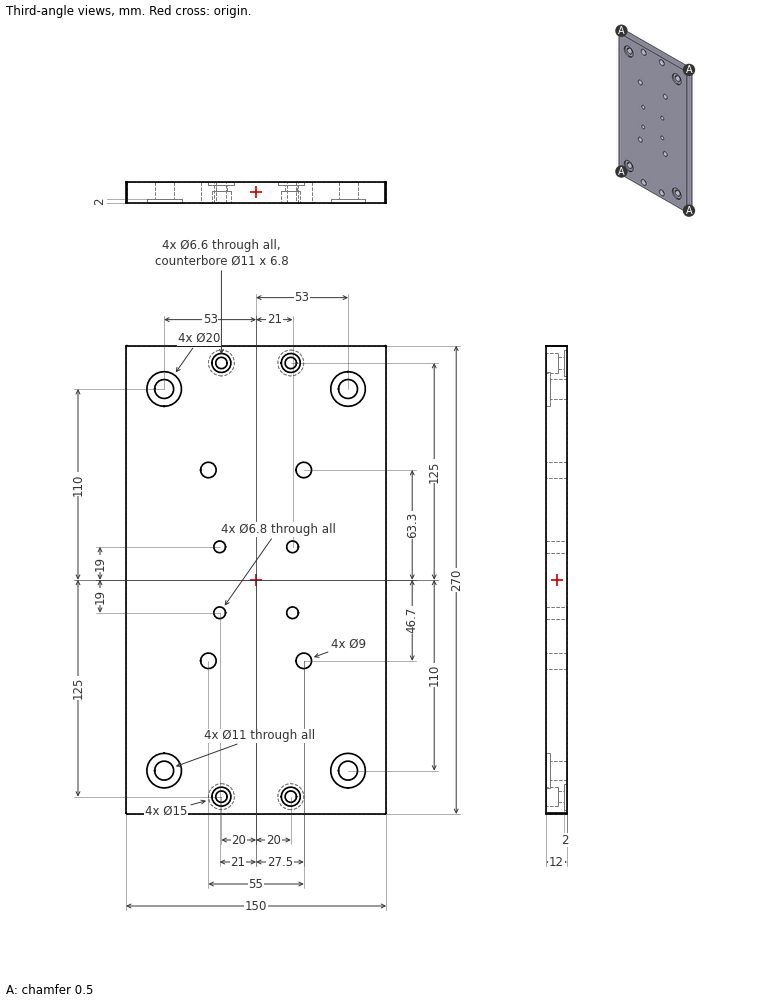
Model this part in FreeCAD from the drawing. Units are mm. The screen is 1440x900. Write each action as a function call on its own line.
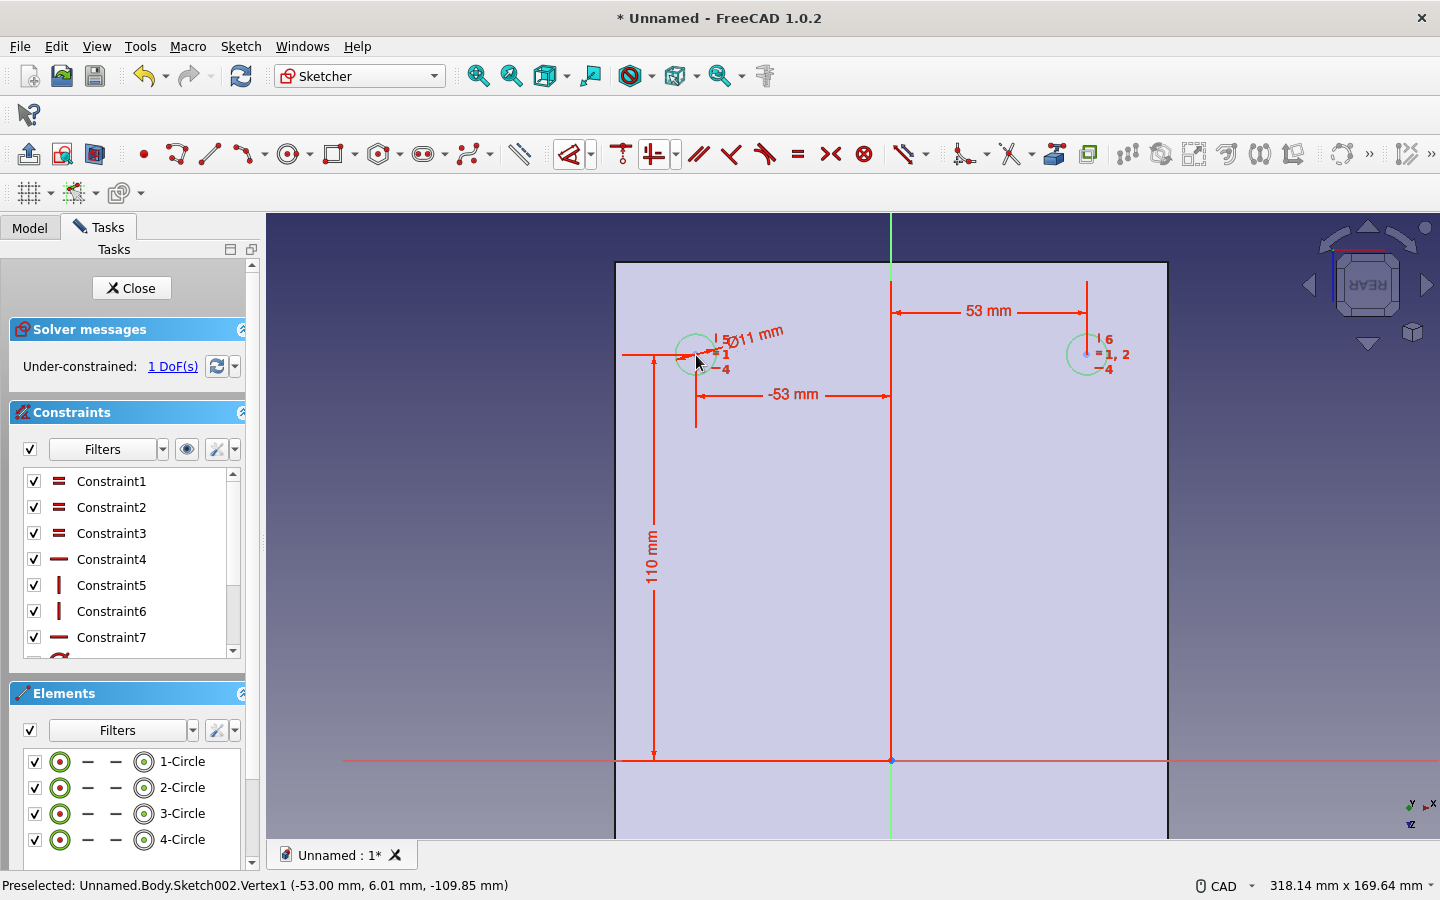
scroll(697, 335, down, 4)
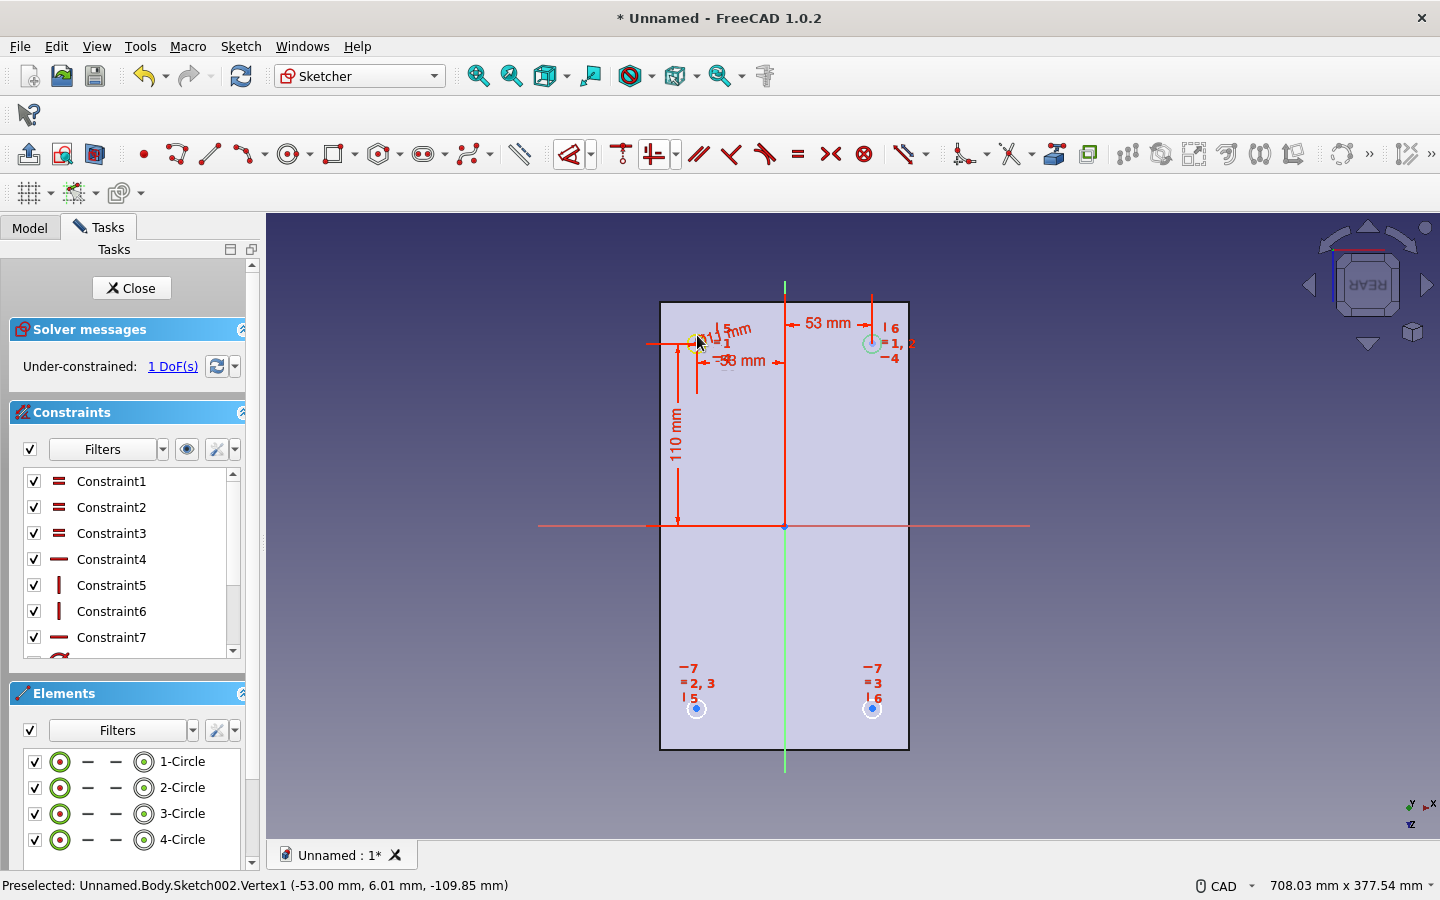
click(697, 709)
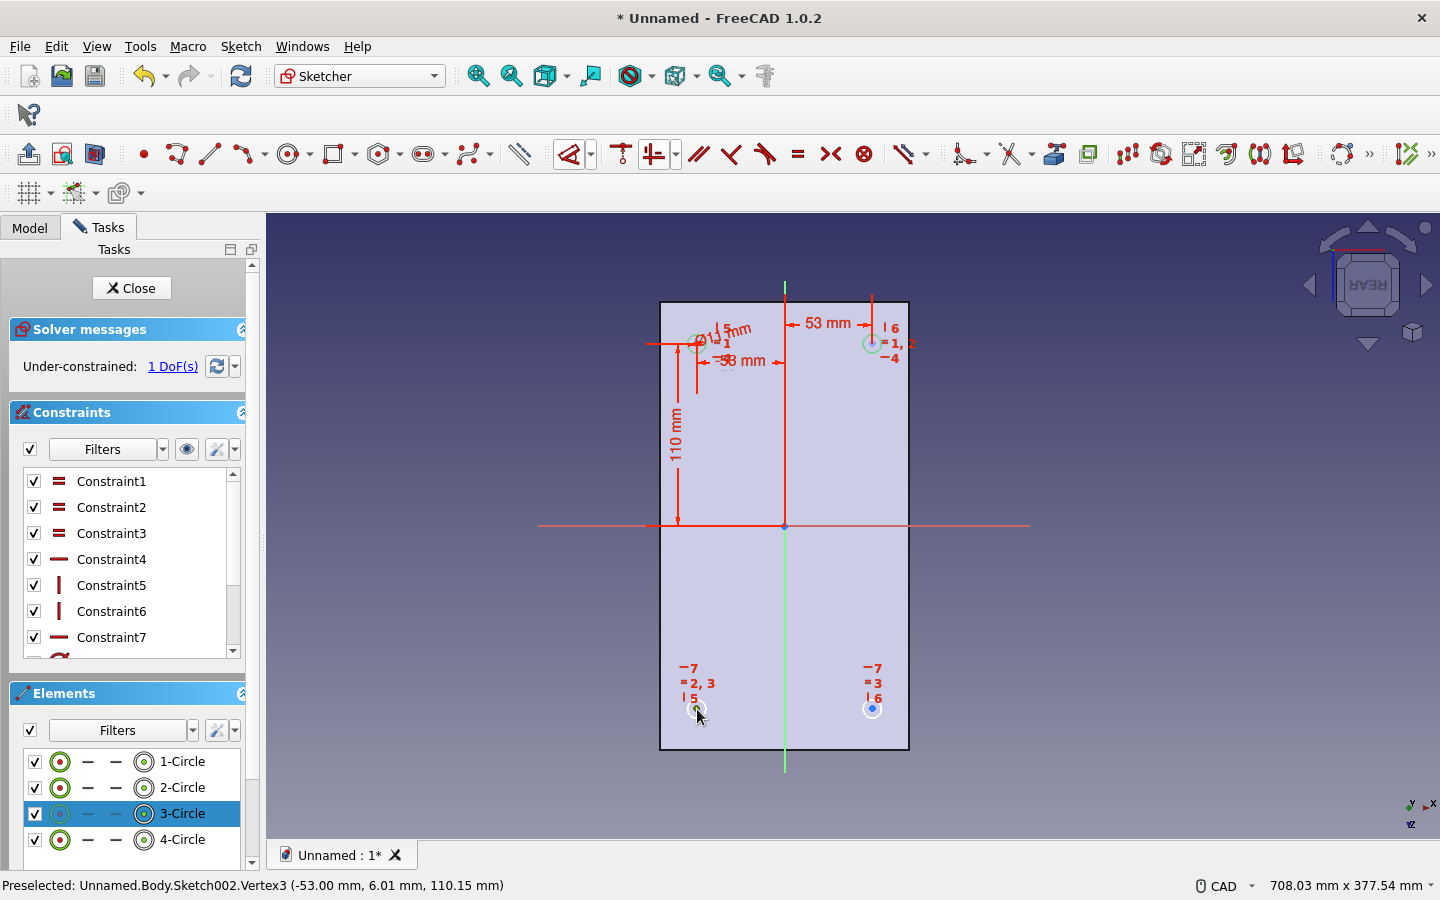
key(i)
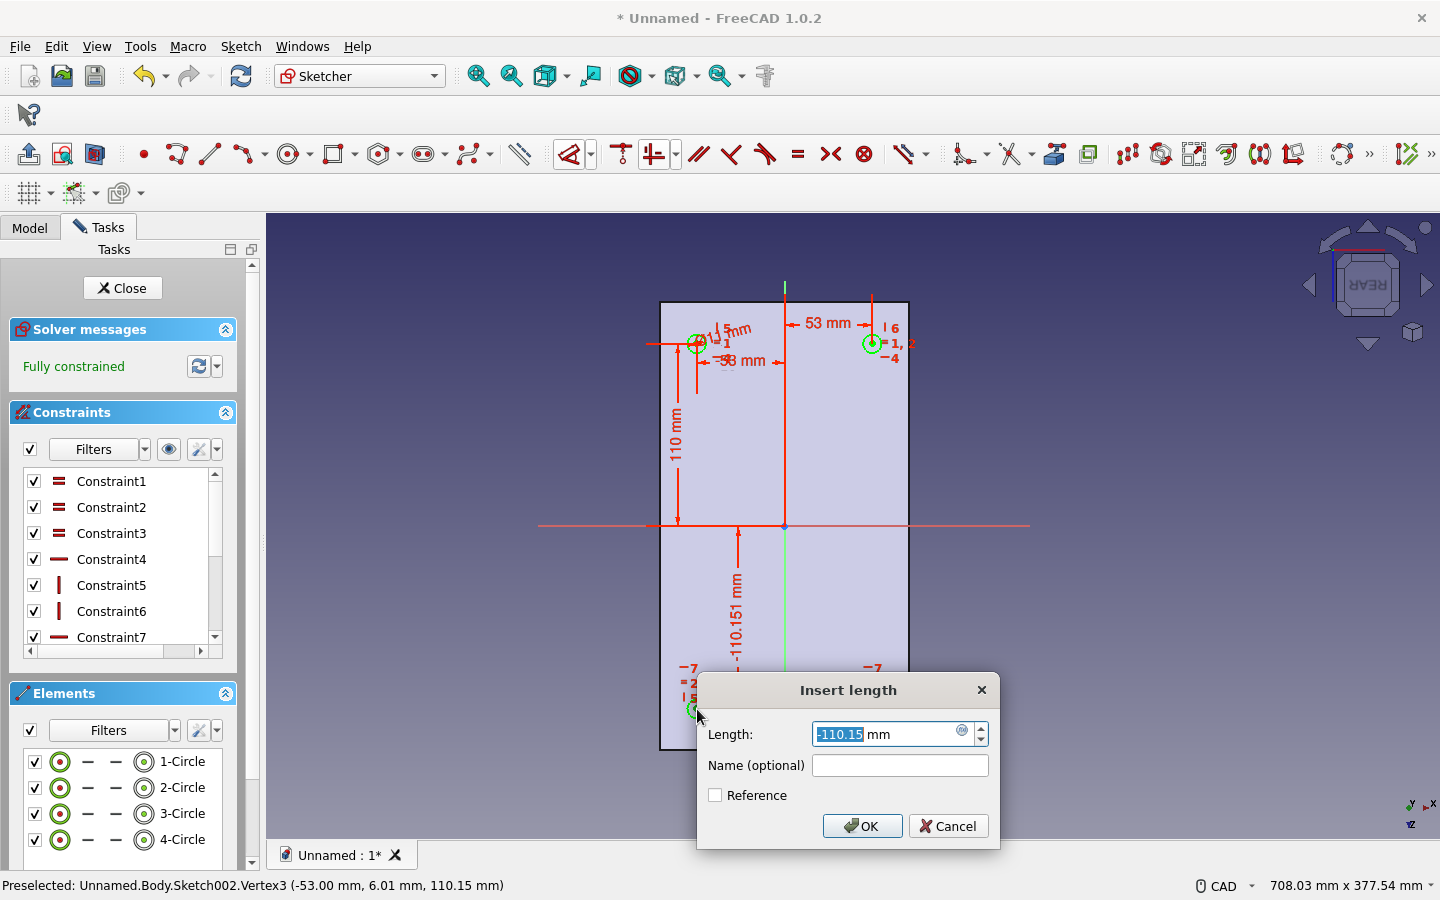
text(-110)
key(Return)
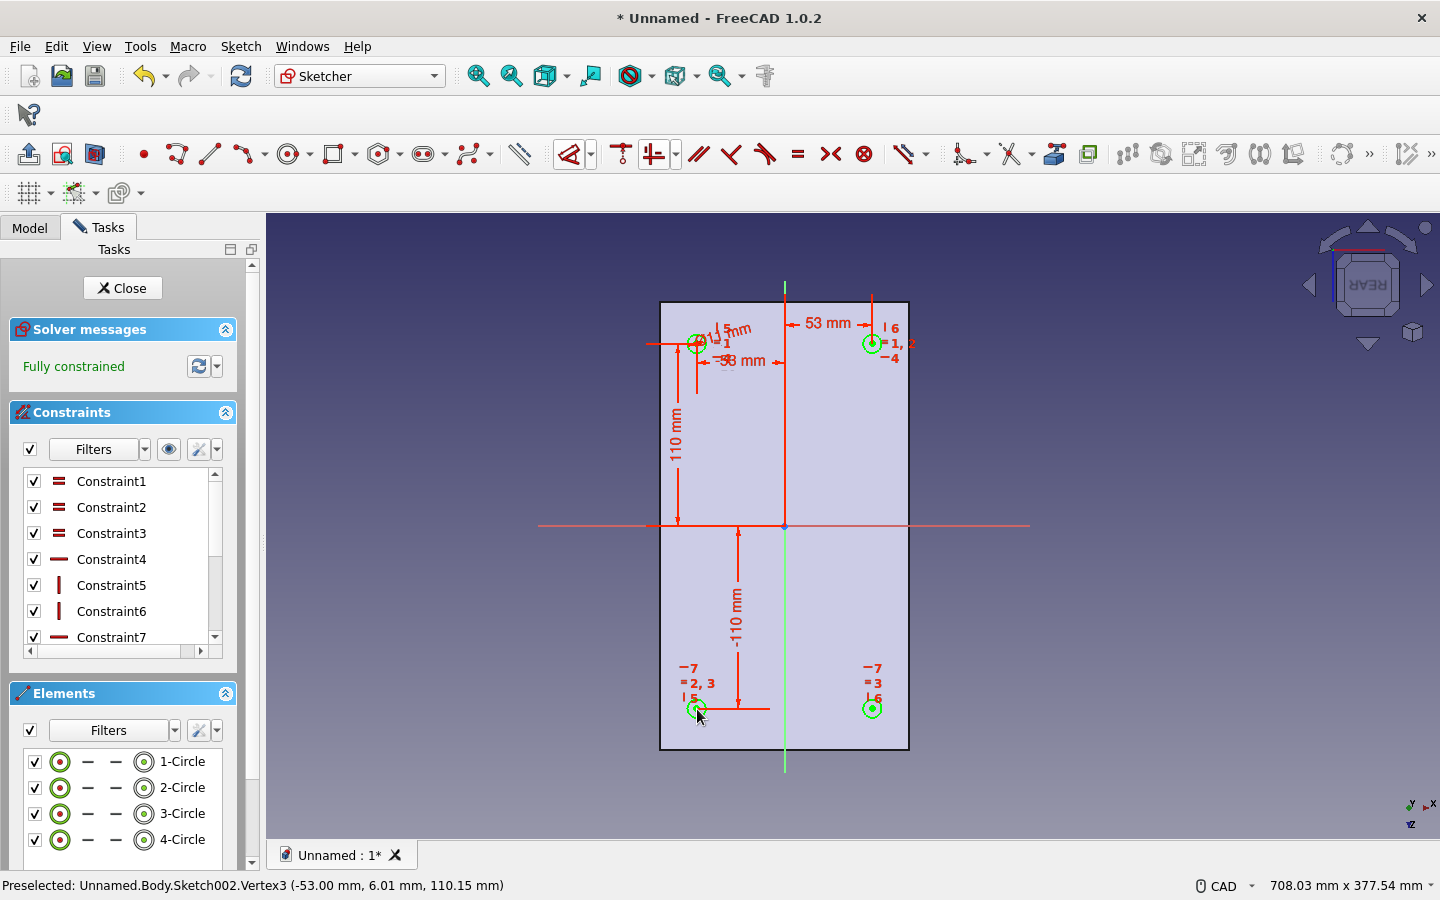
click(123, 288)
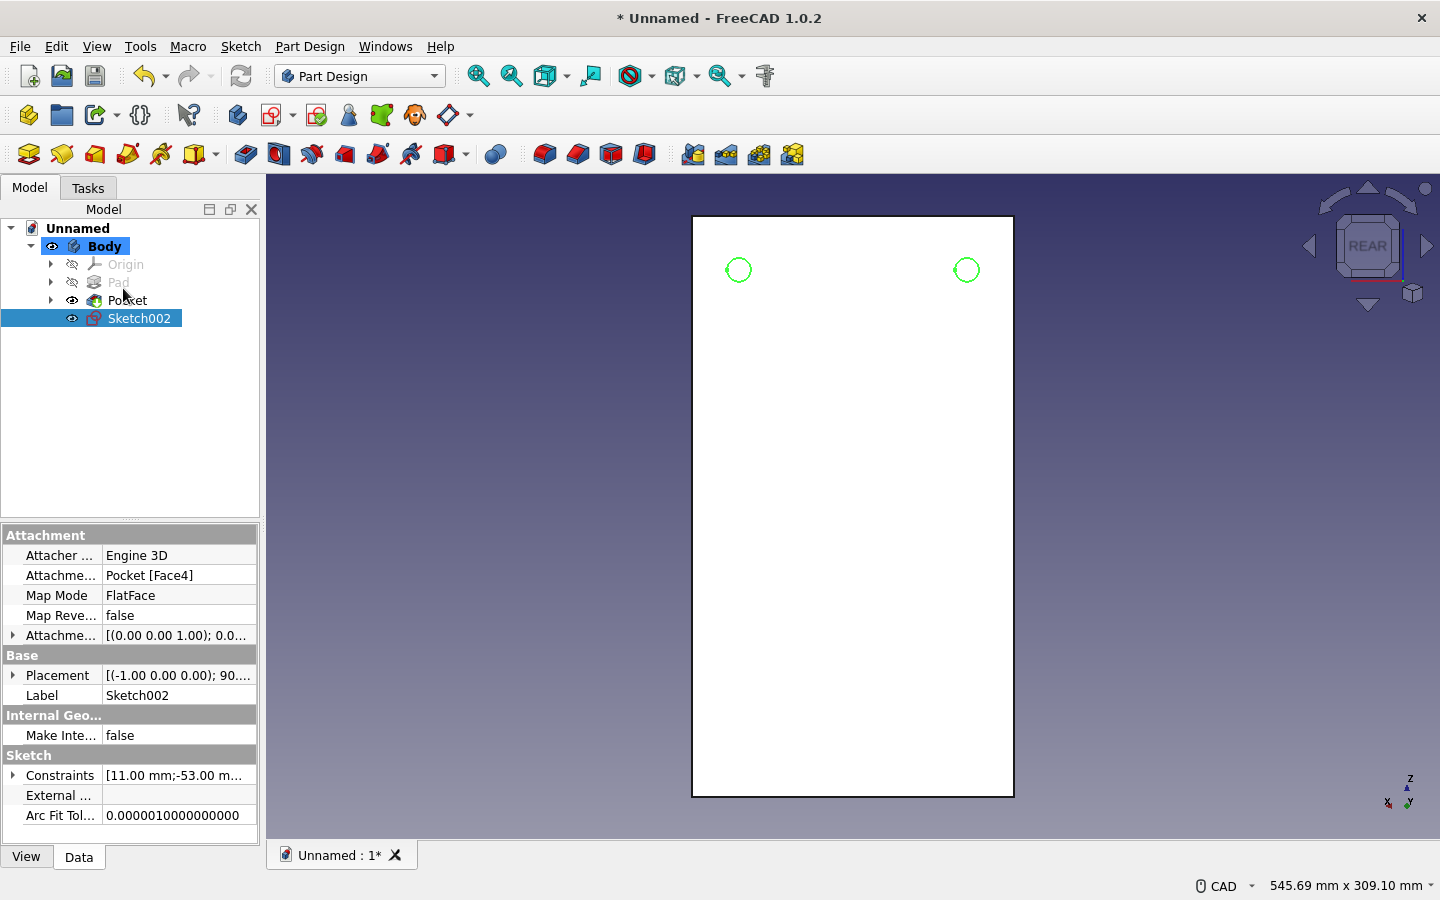
click(279, 154)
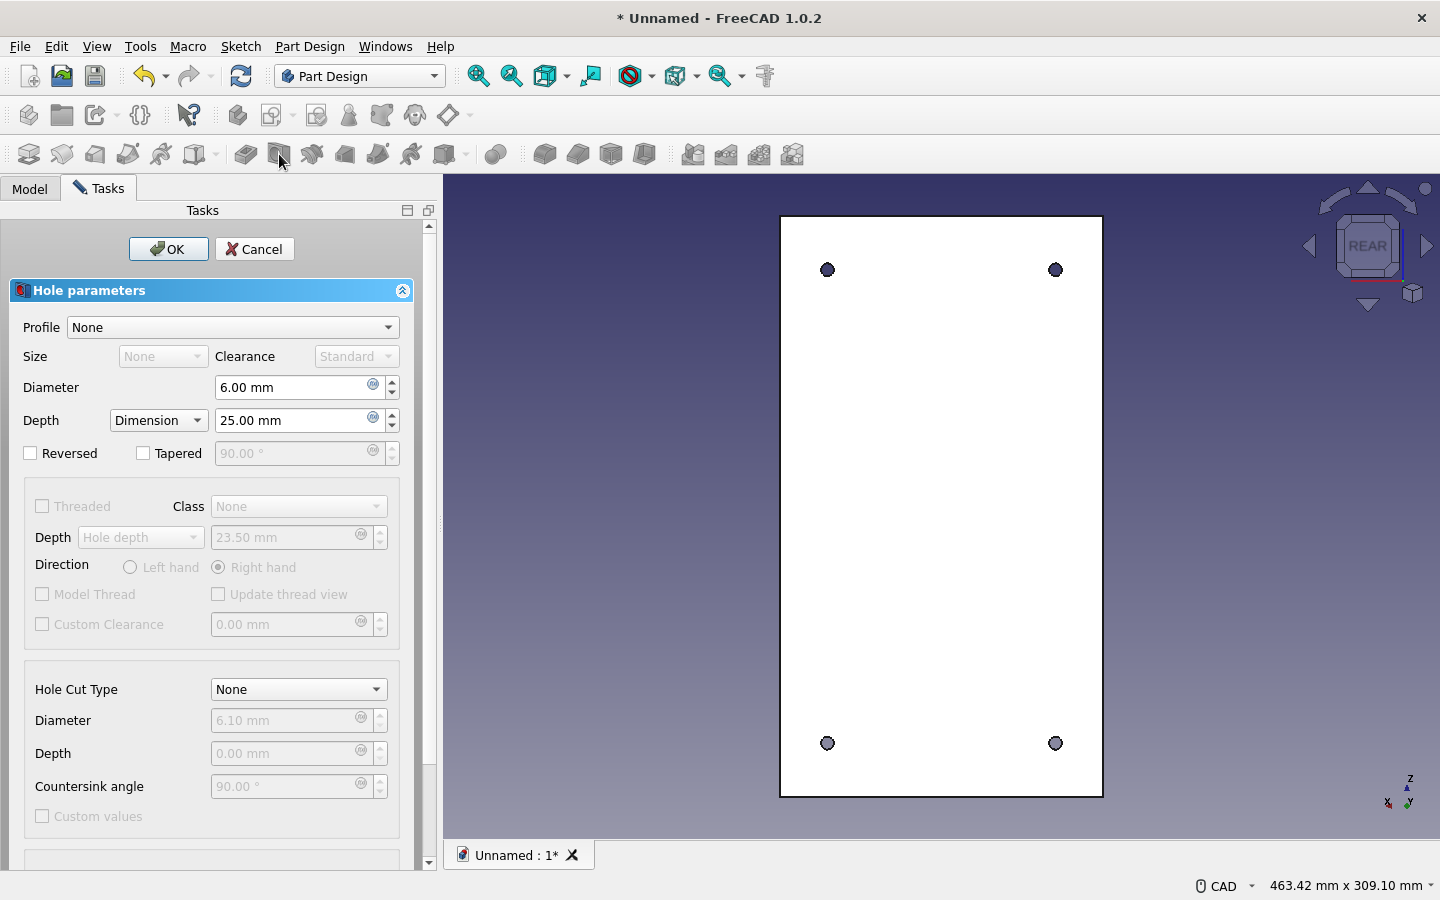
triple_click(300, 388)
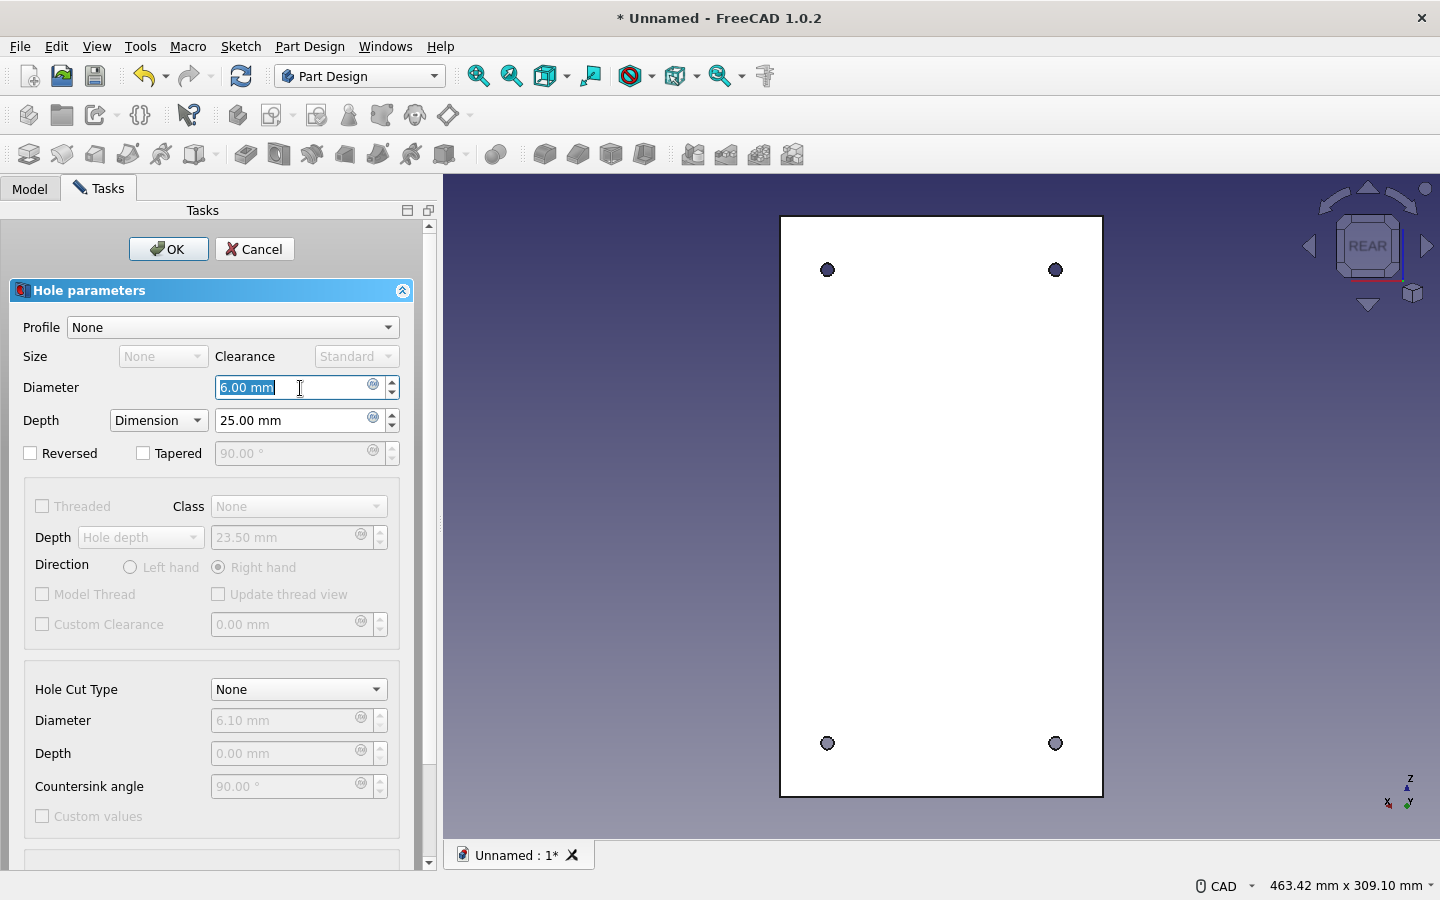
text(11)
key(Tab)